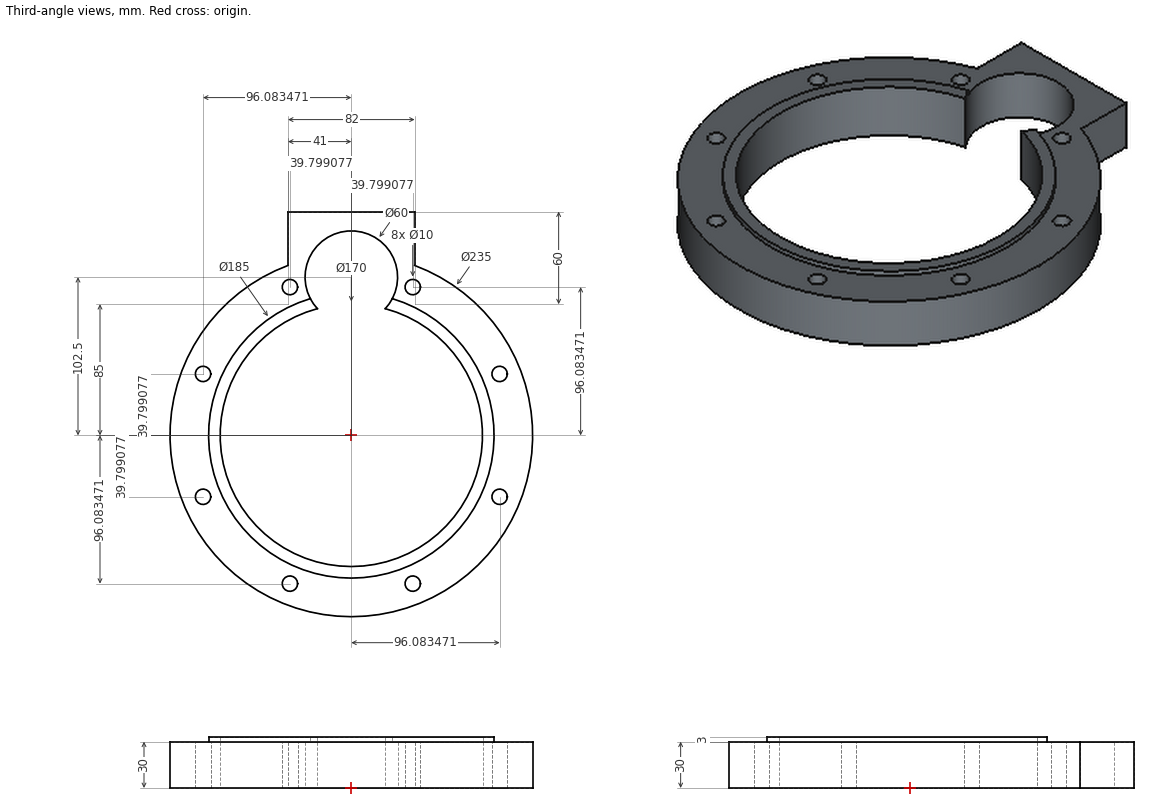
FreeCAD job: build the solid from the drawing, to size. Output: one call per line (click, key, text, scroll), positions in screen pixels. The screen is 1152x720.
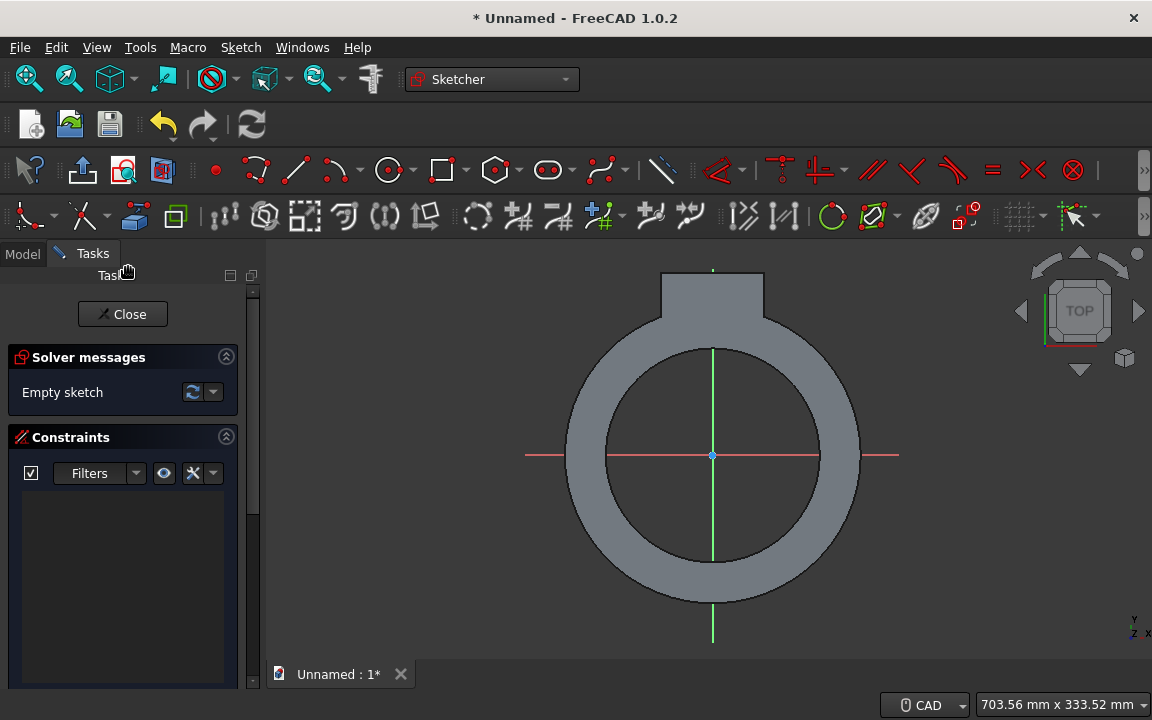
click(164, 170)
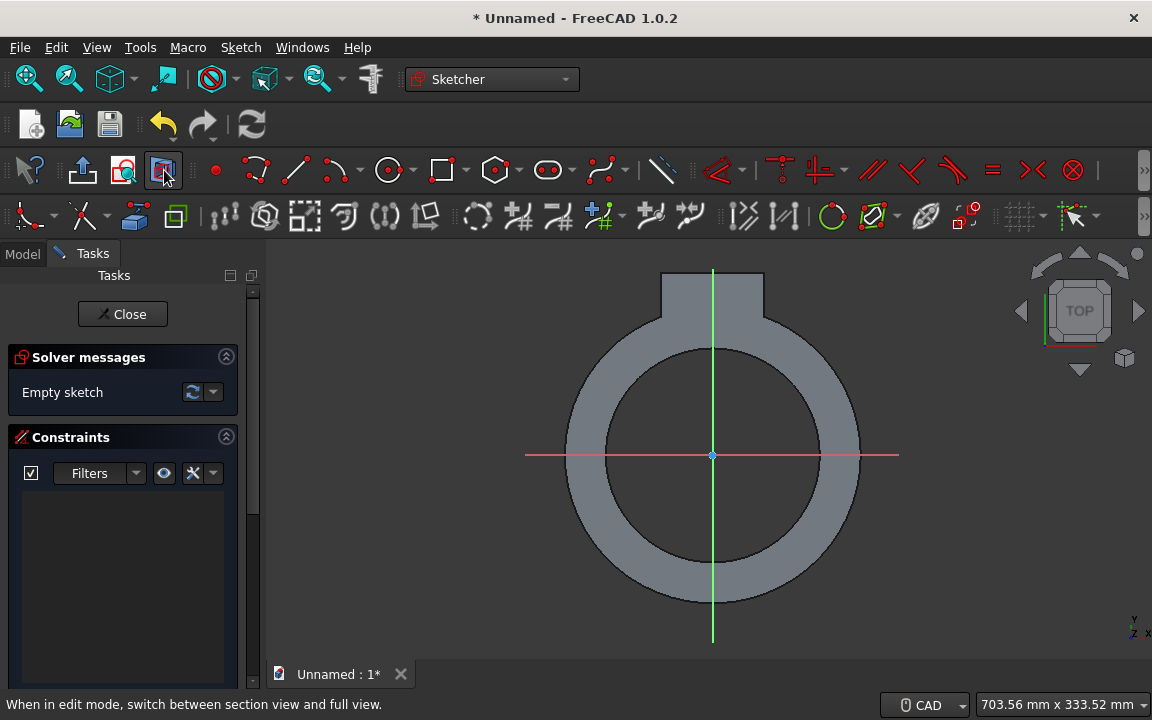
click(390, 170)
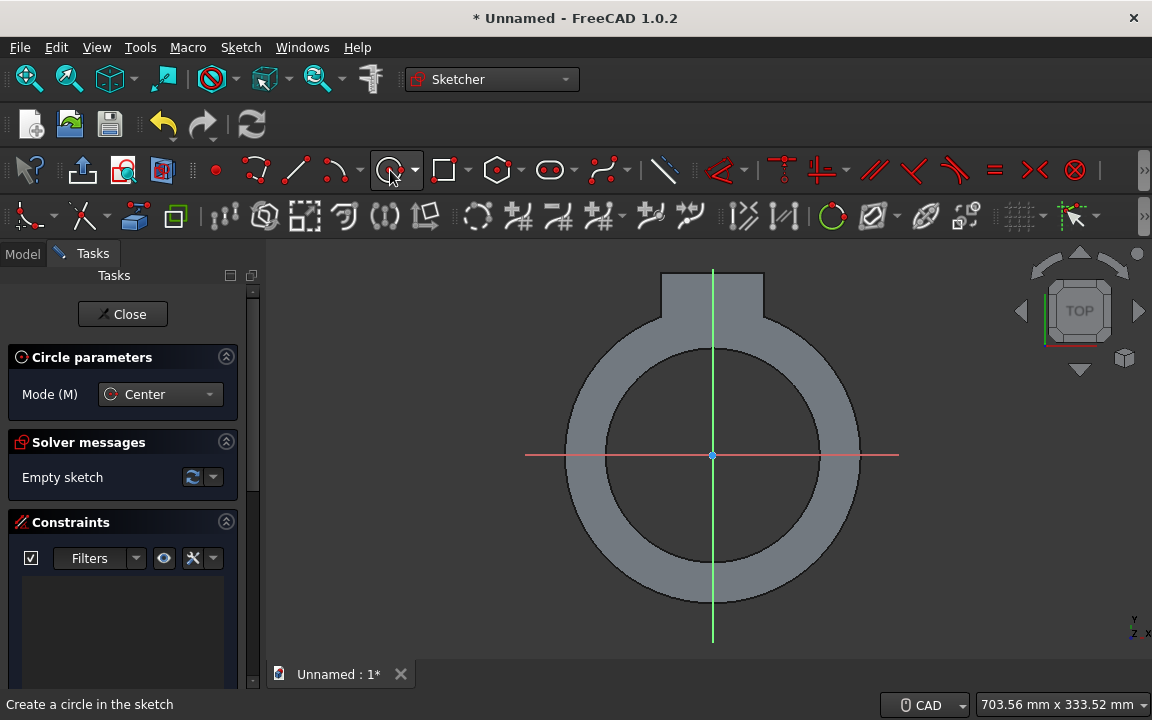
scroll(763, 334, up, 7)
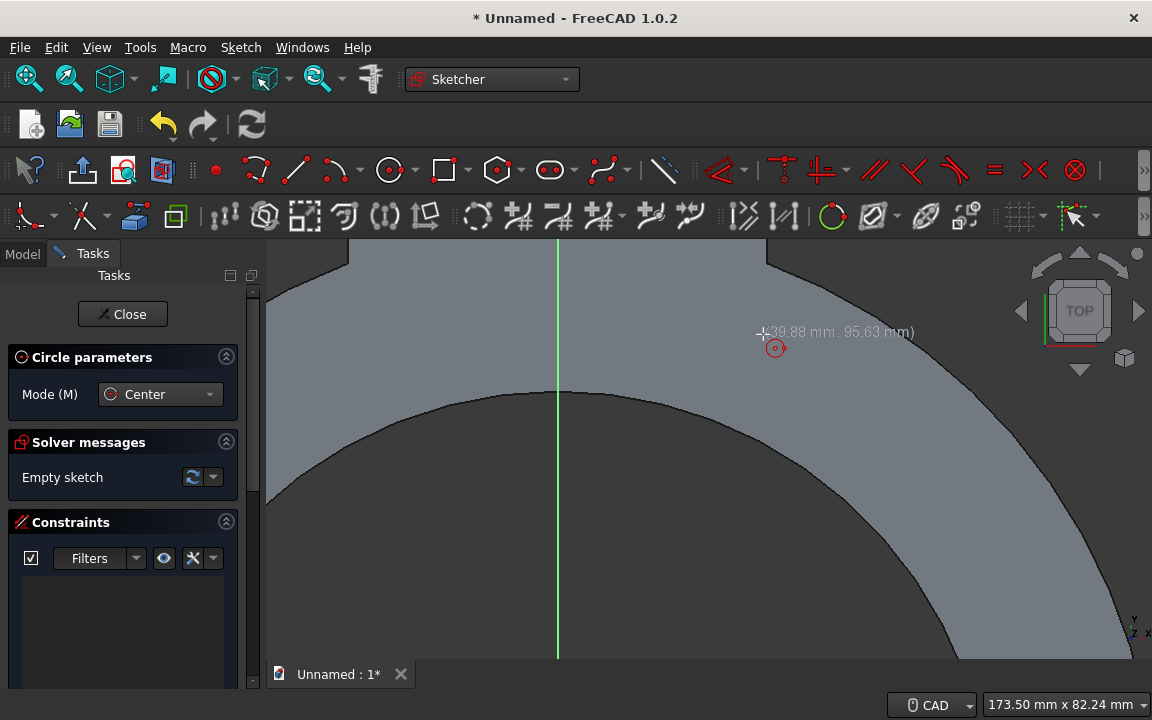
scroll(668, 326, down, 7)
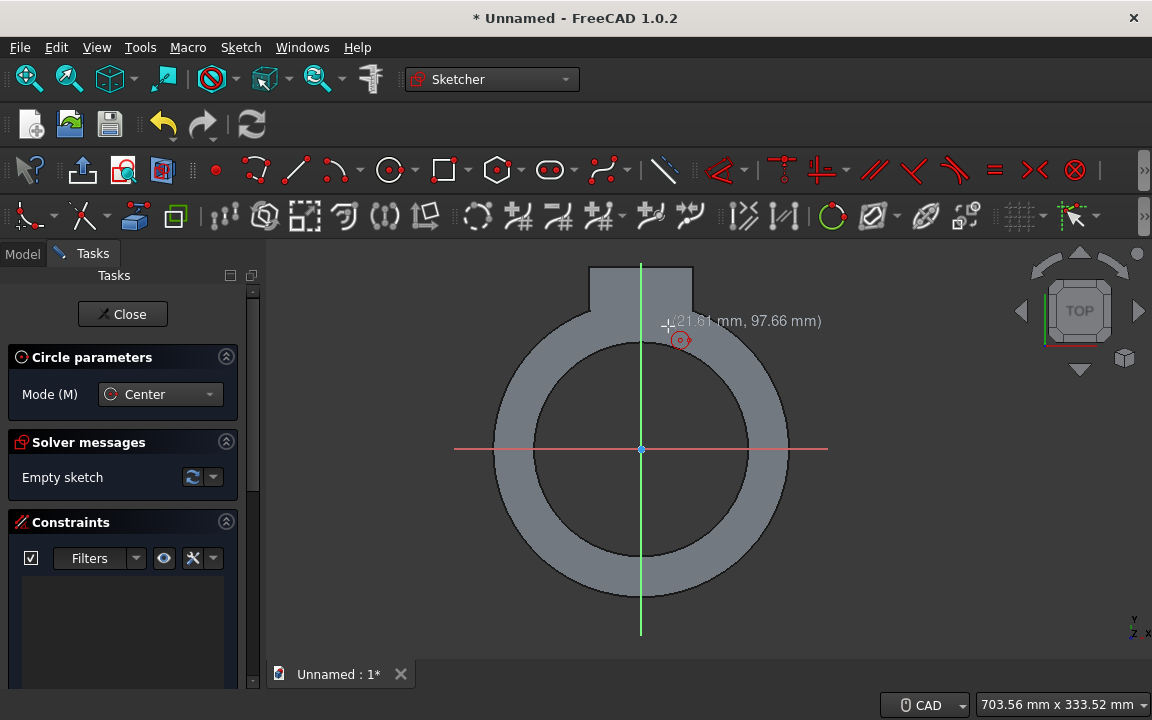
click(691, 328)
move(696, 324)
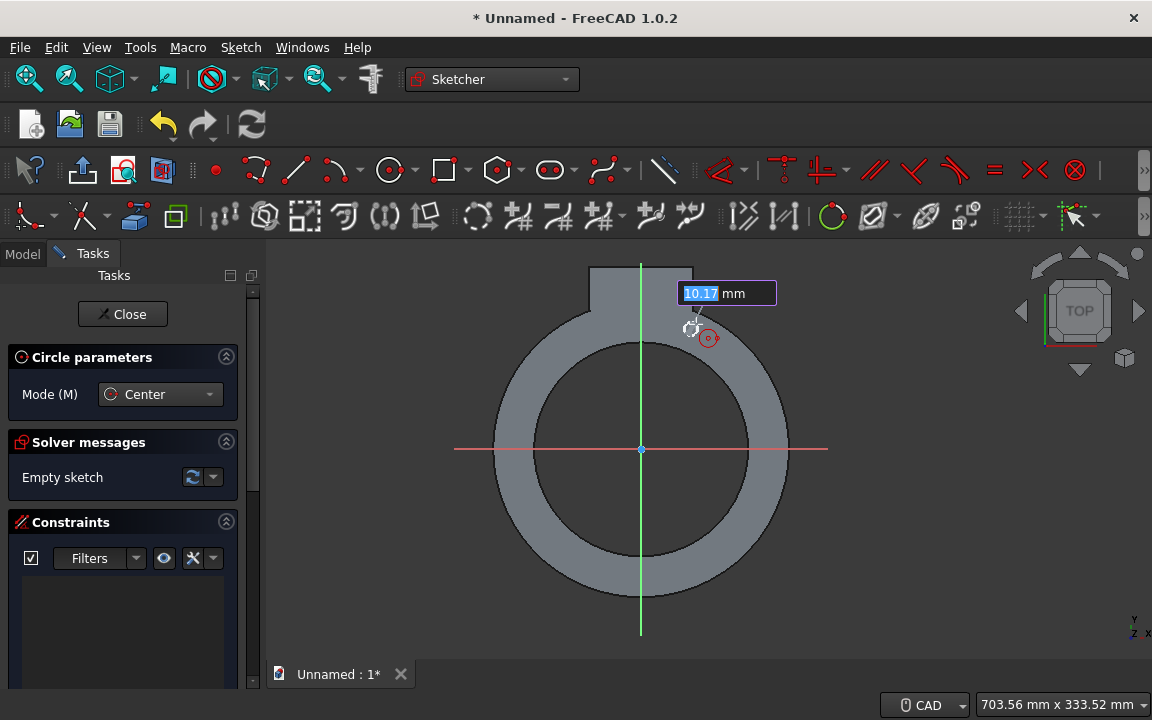
text(10)
key(Return)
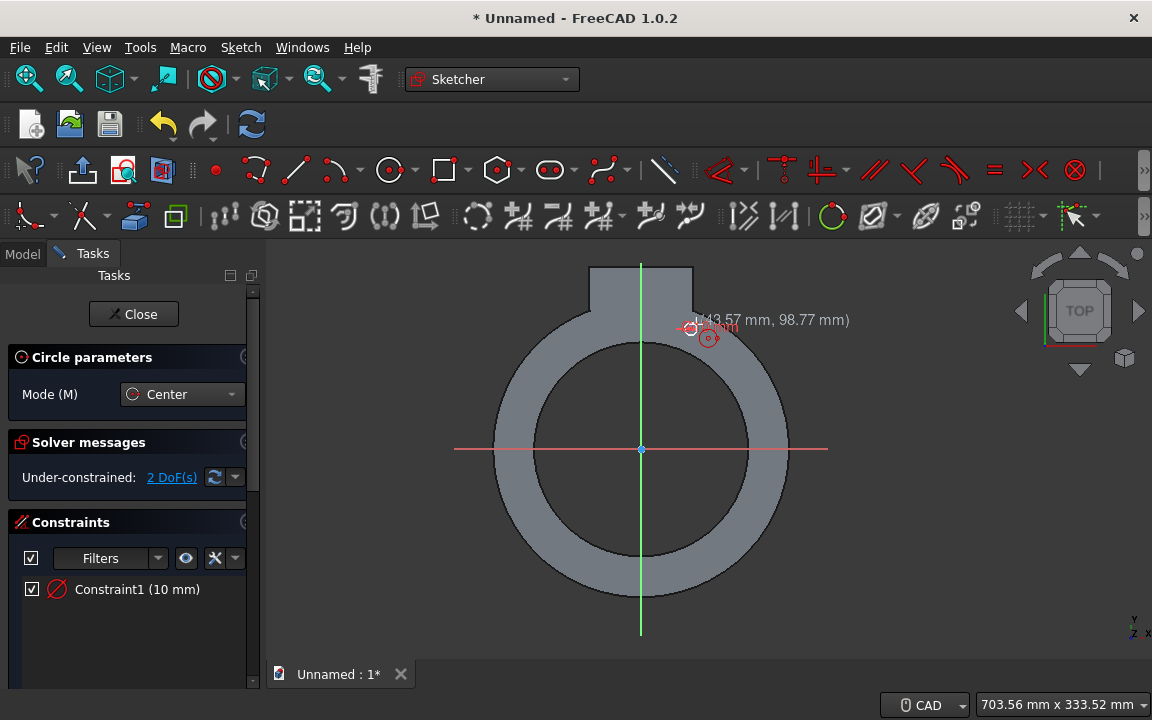
scroll(591, 328, up, 7)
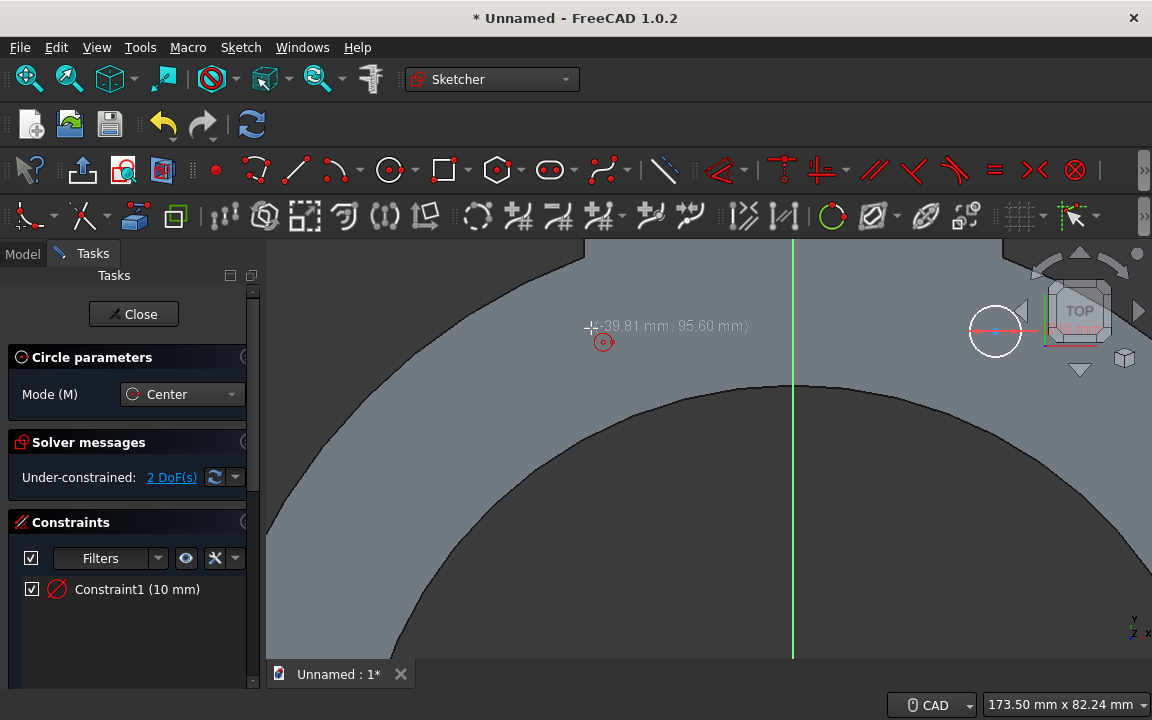
scroll(591, 328, down, 7)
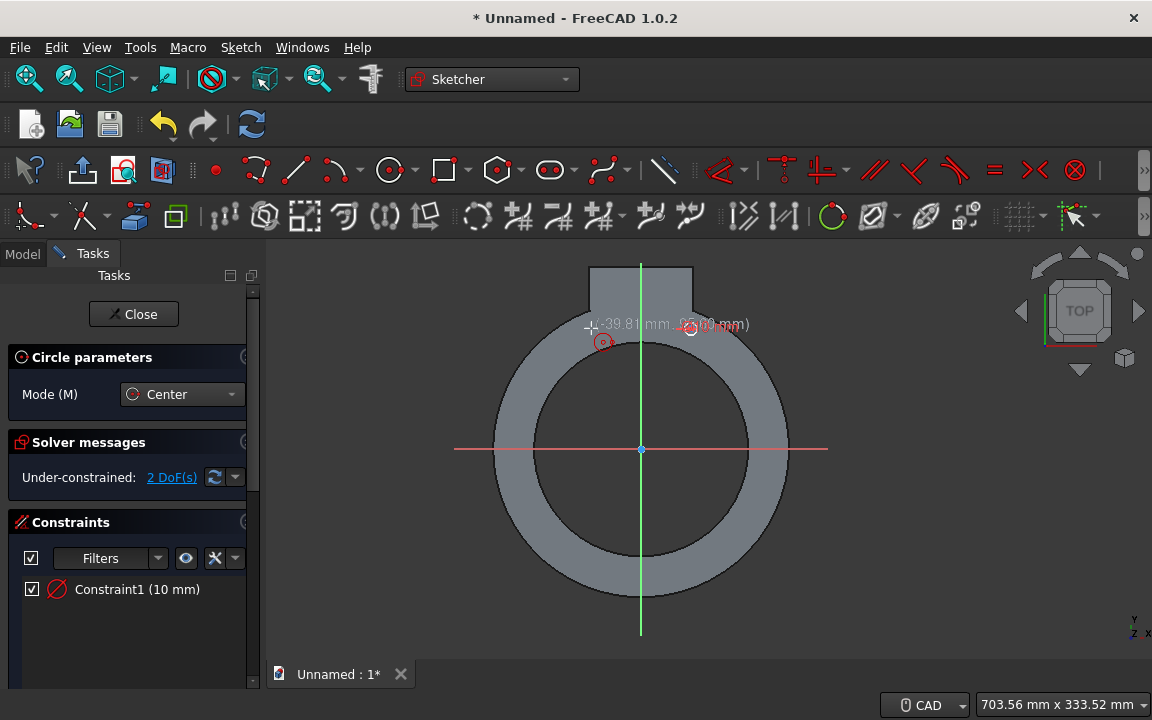
click(591, 328)
move(595, 324)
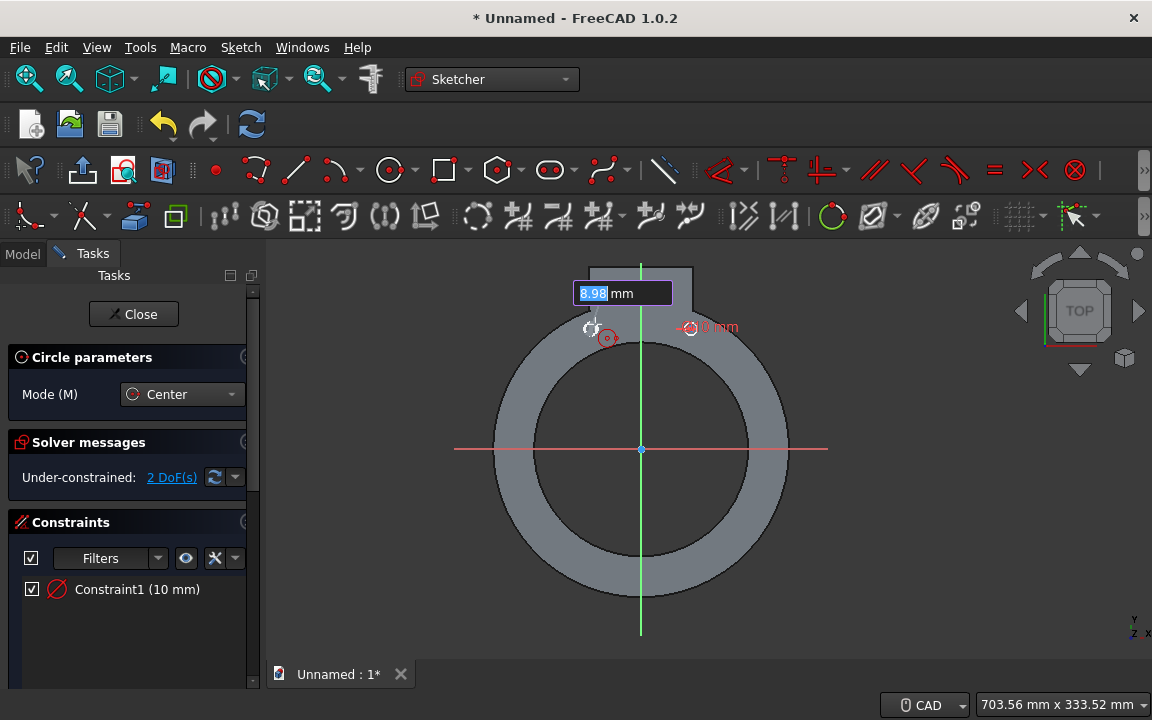
text(10)
key(Return)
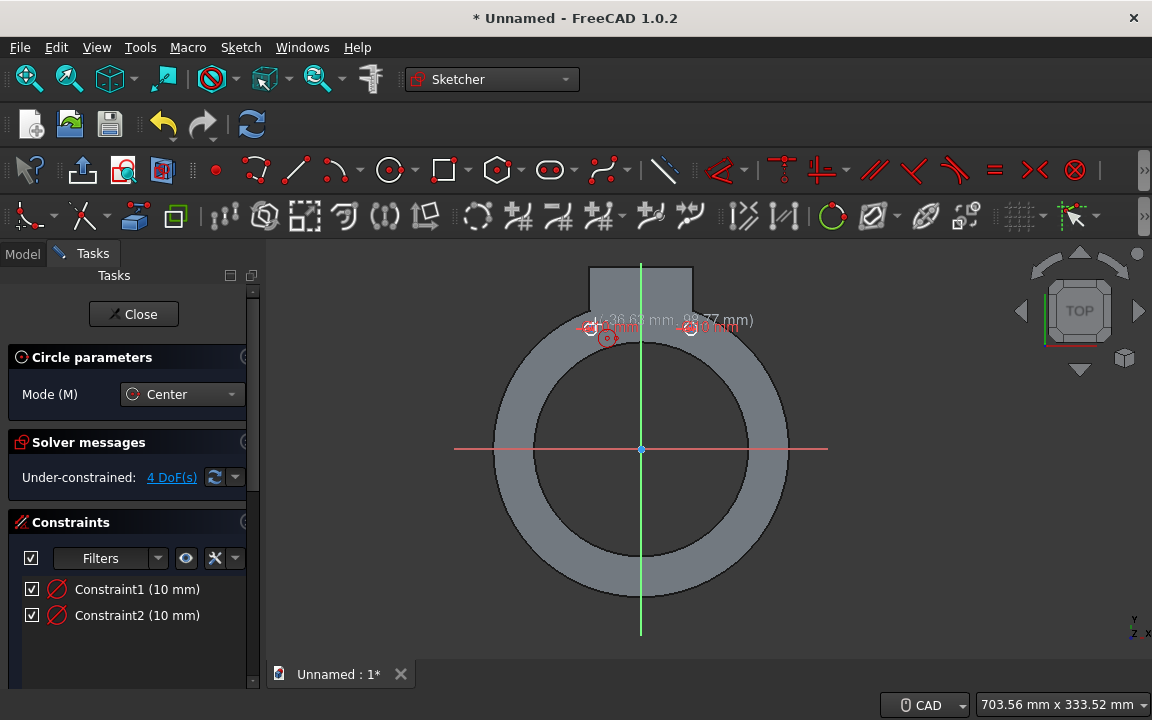
scroll(520, 399, up, 7)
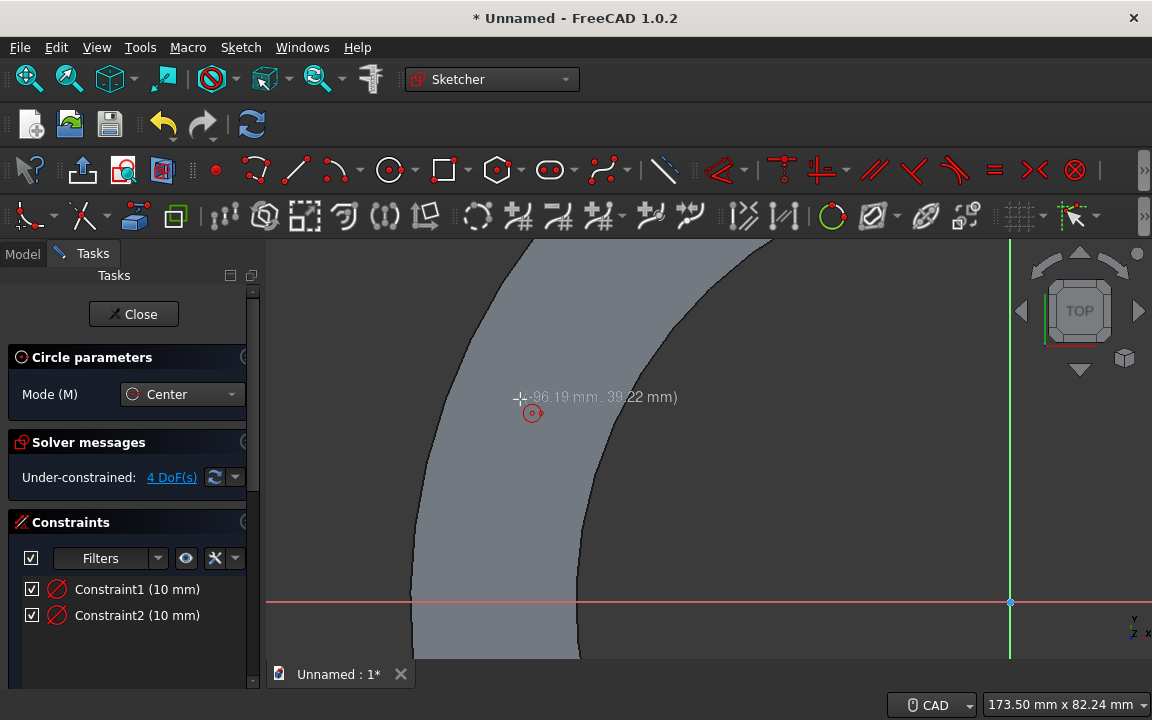
scroll(519, 399, down, 7)